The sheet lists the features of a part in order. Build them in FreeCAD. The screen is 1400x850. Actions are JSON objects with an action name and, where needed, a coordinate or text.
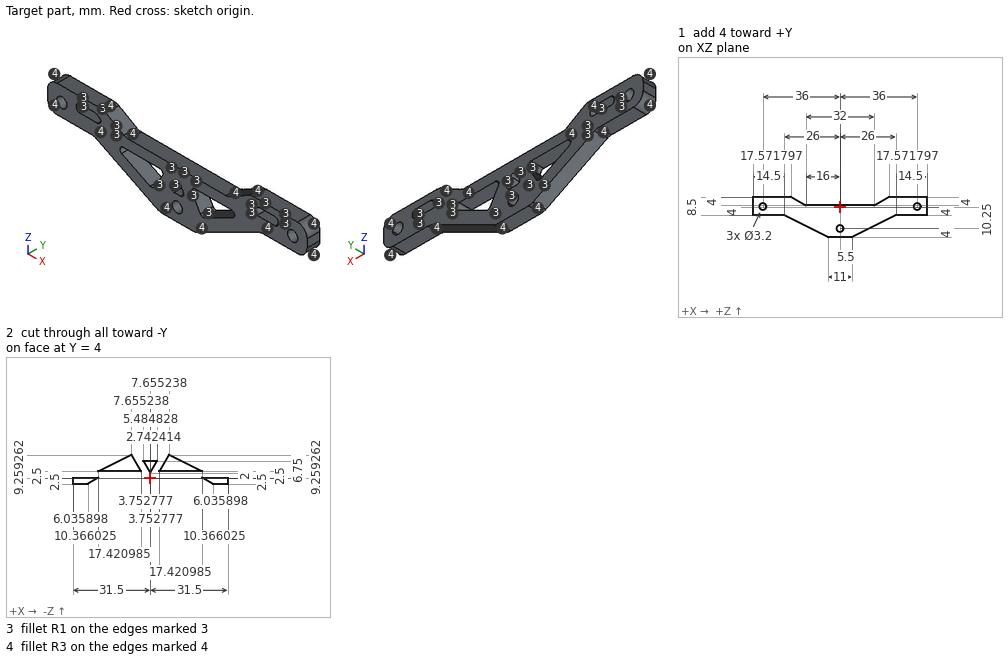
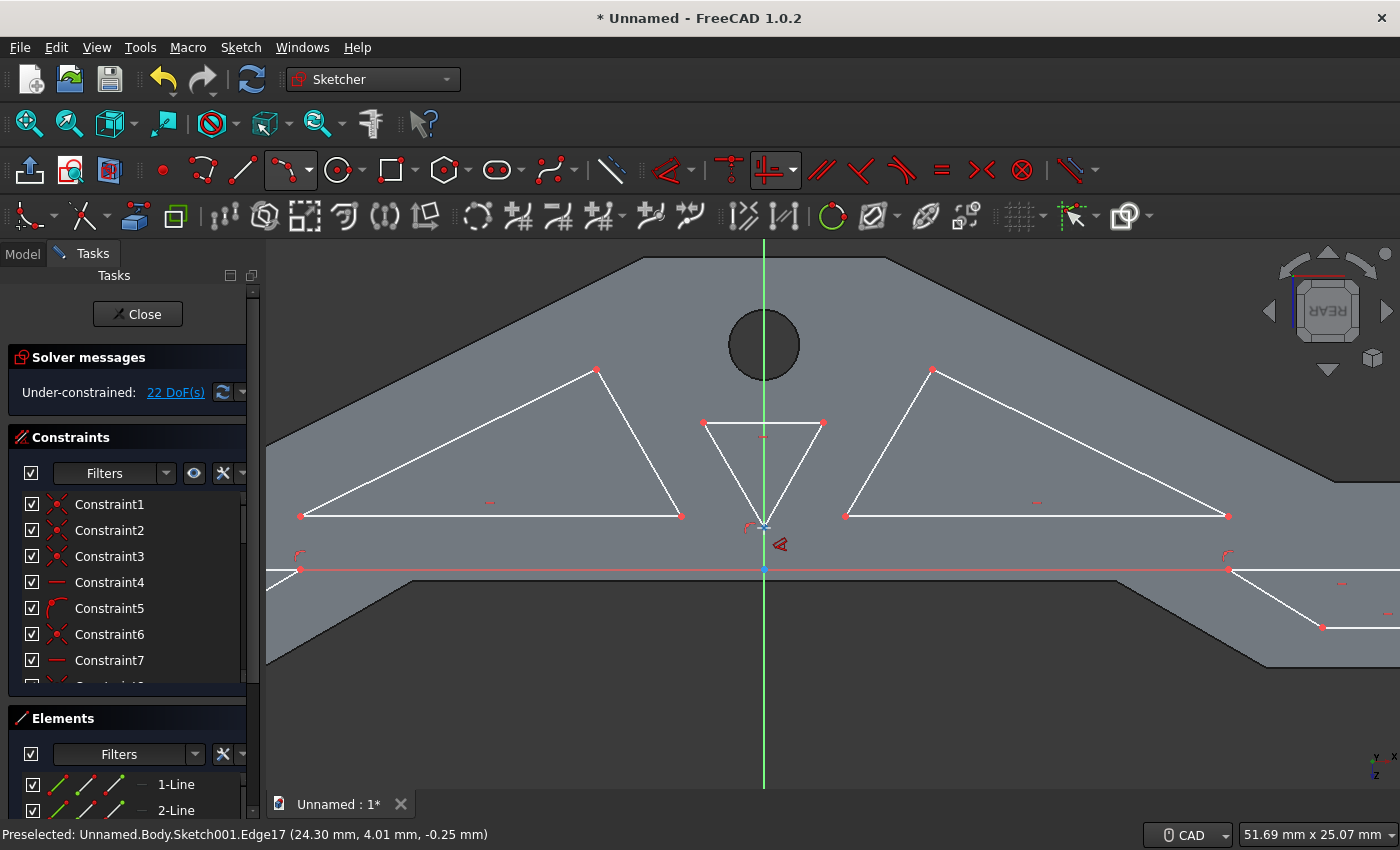
{"action": "left_click", "coordinate": [764, 527]}
{"action": "left_click", "coordinate": [798, 549]}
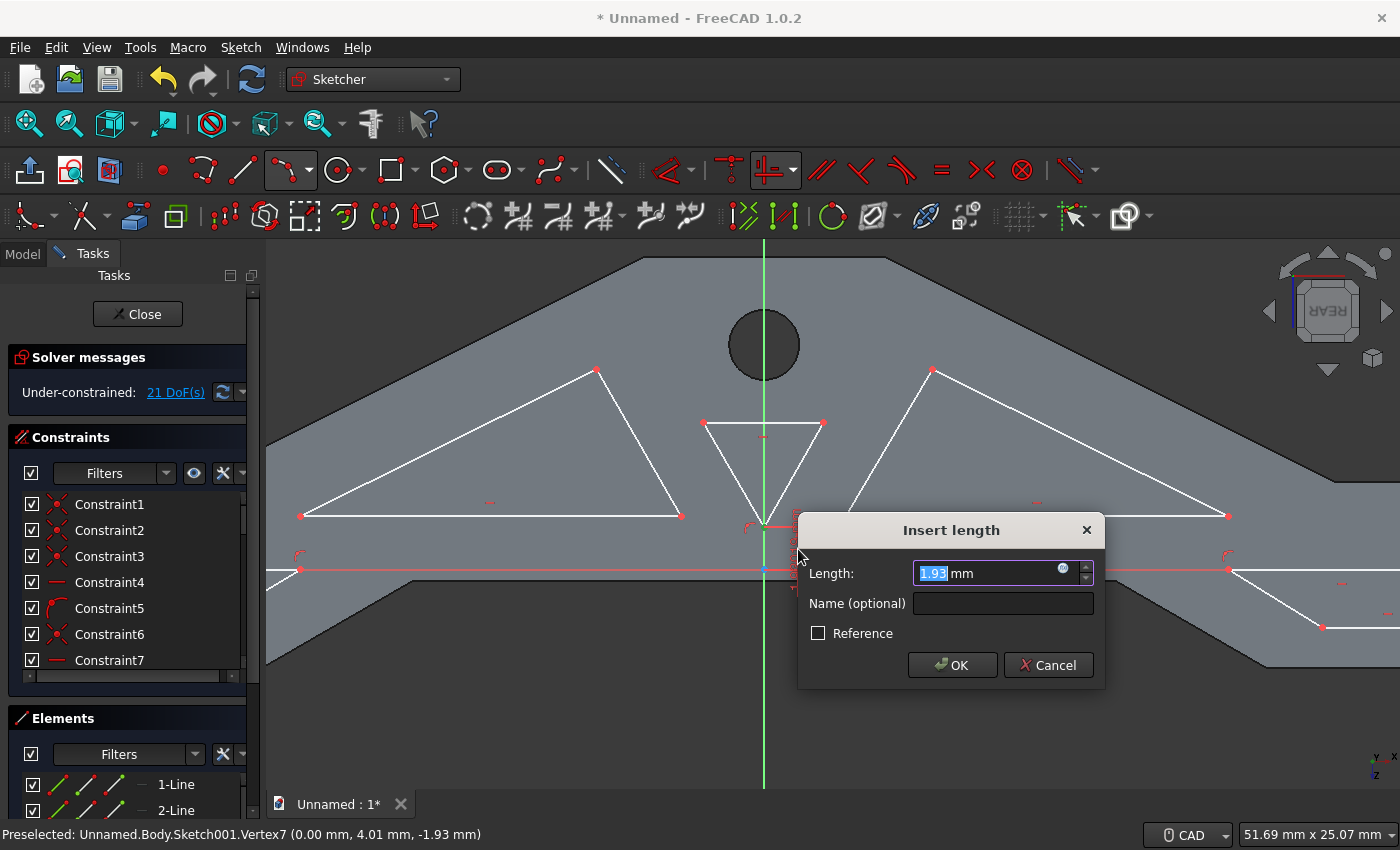
{"action": "type", "text": "2"}
{"action": "key", "text": "Return"}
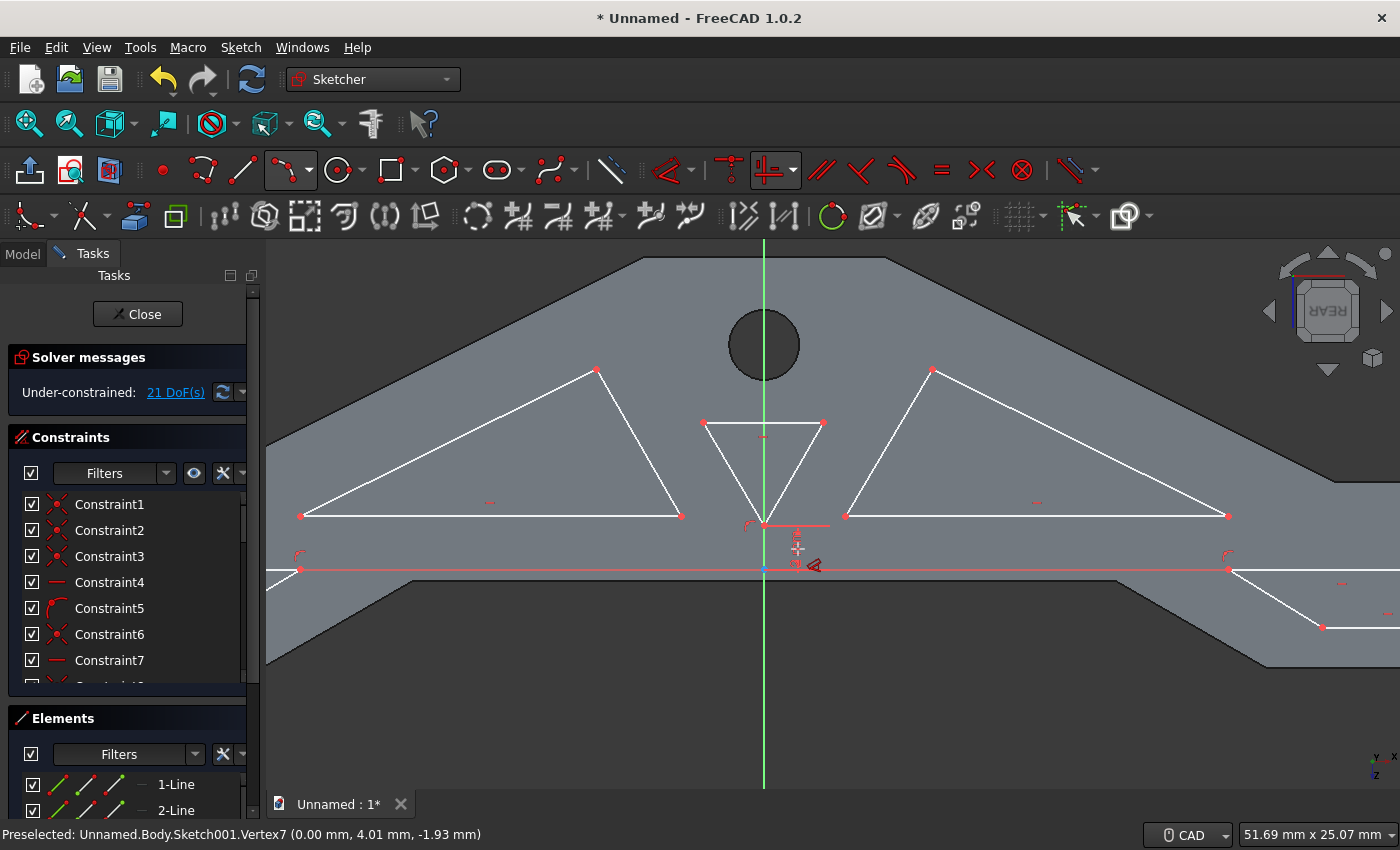
{"action": "scroll", "coordinate": [765, 529], "scroll_direction": "down", "scroll_amount": 4}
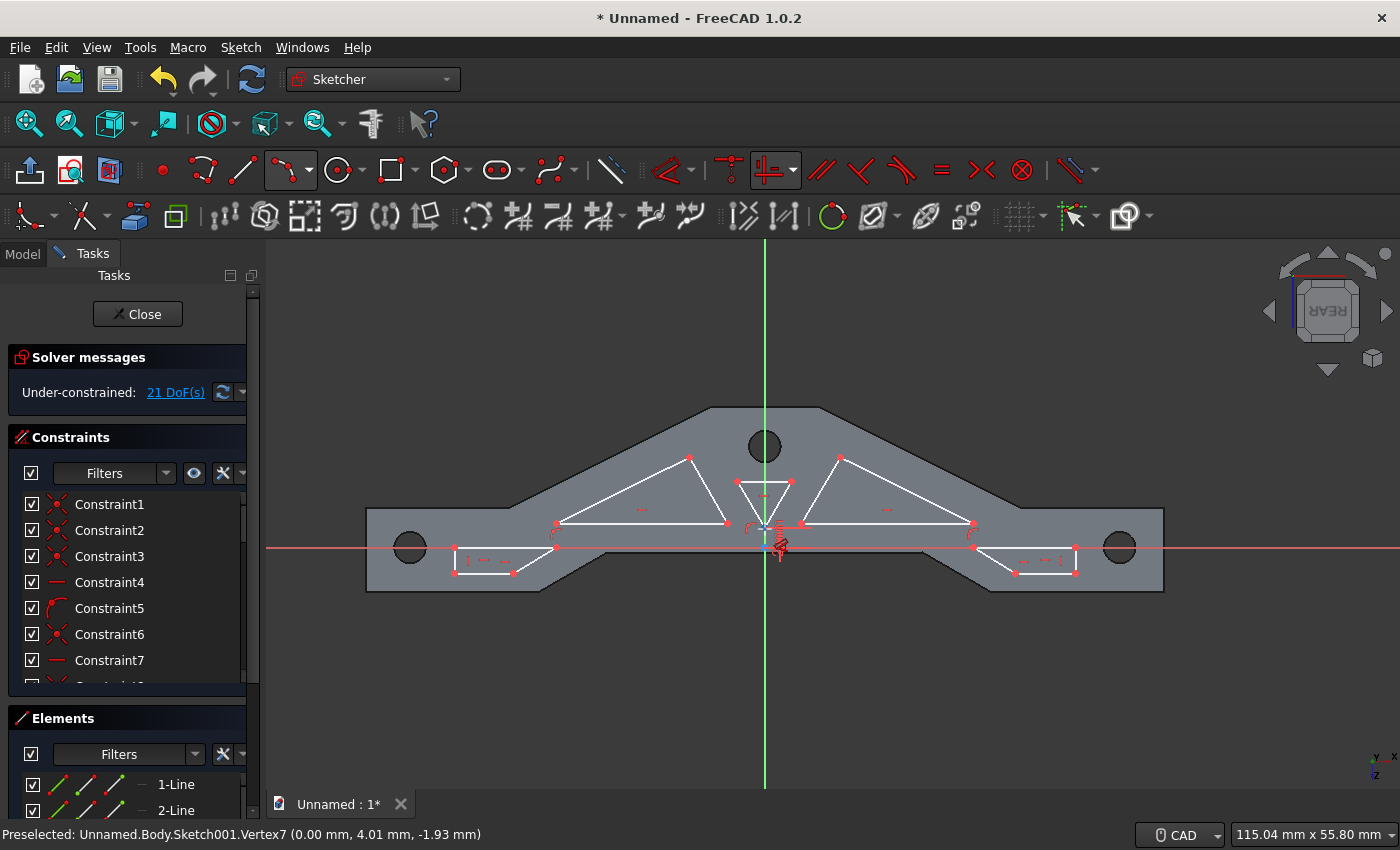
{"action": "scroll", "coordinate": [455, 555], "scroll_direction": "up", "scroll_amount": 3}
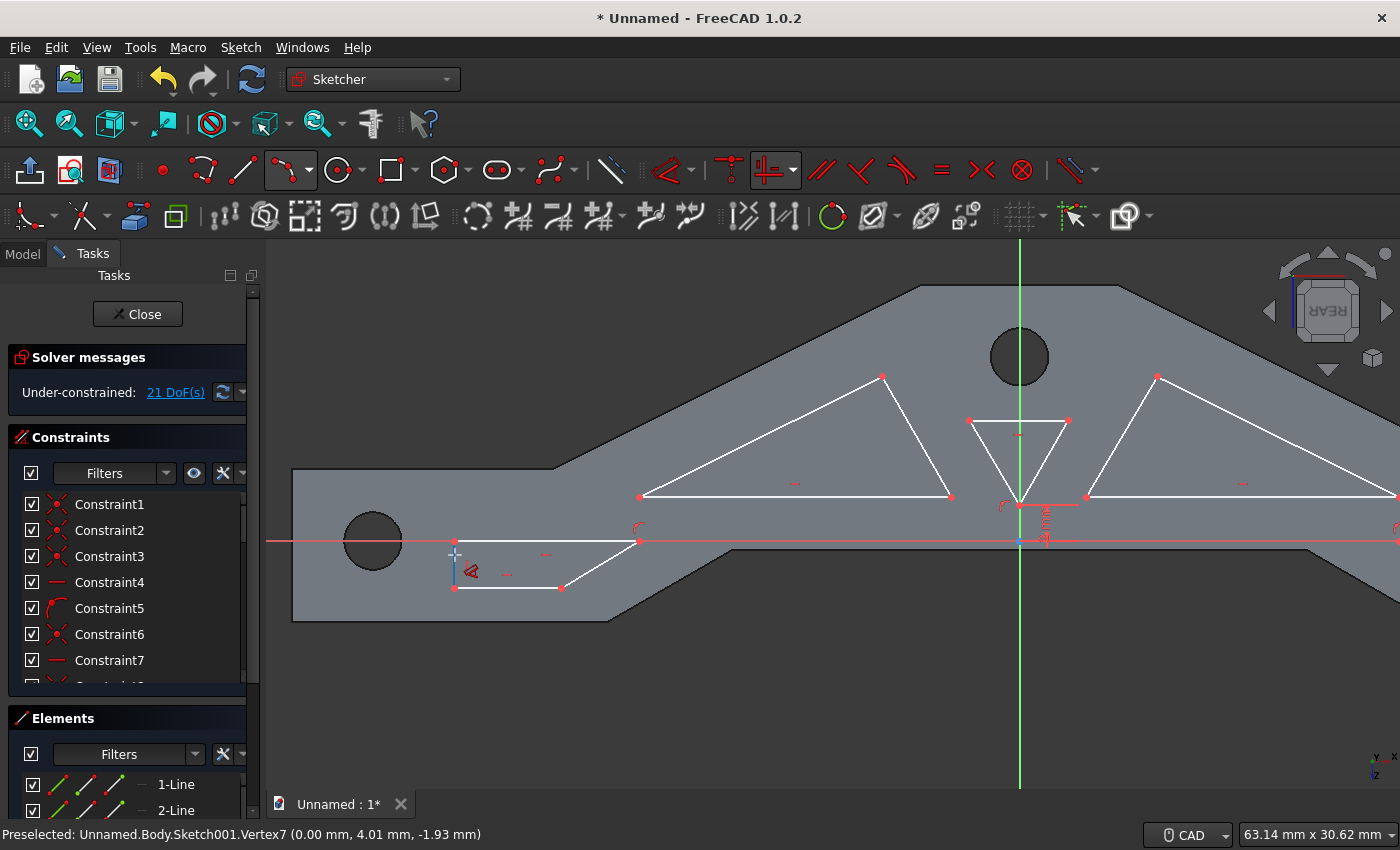
{"action": "left_click", "coordinate": [454, 555]}
{"action": "left_click", "coordinate": [420, 565]}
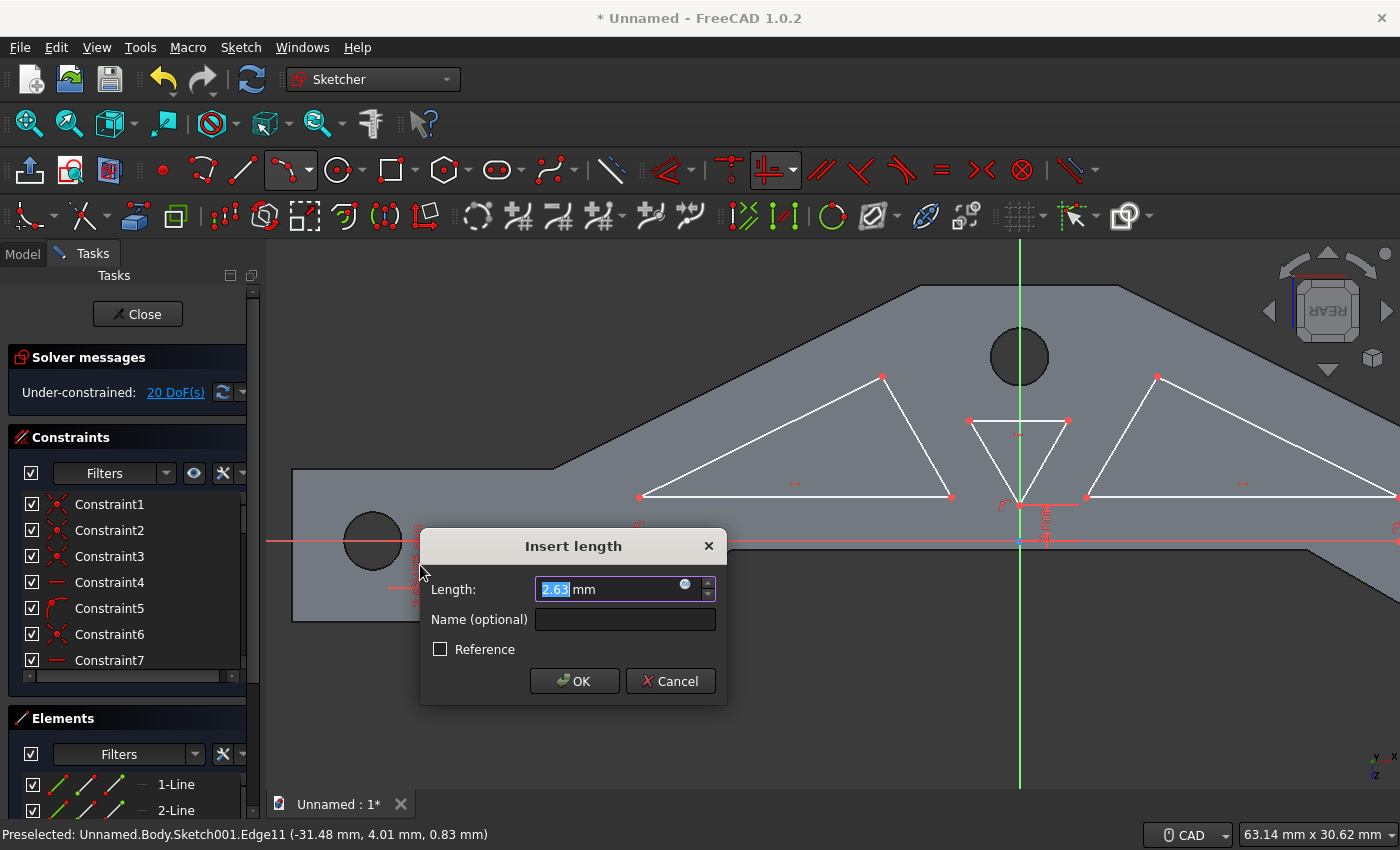
{"action": "type", "text": "2.5"}
{"action": "key", "text": "Return"}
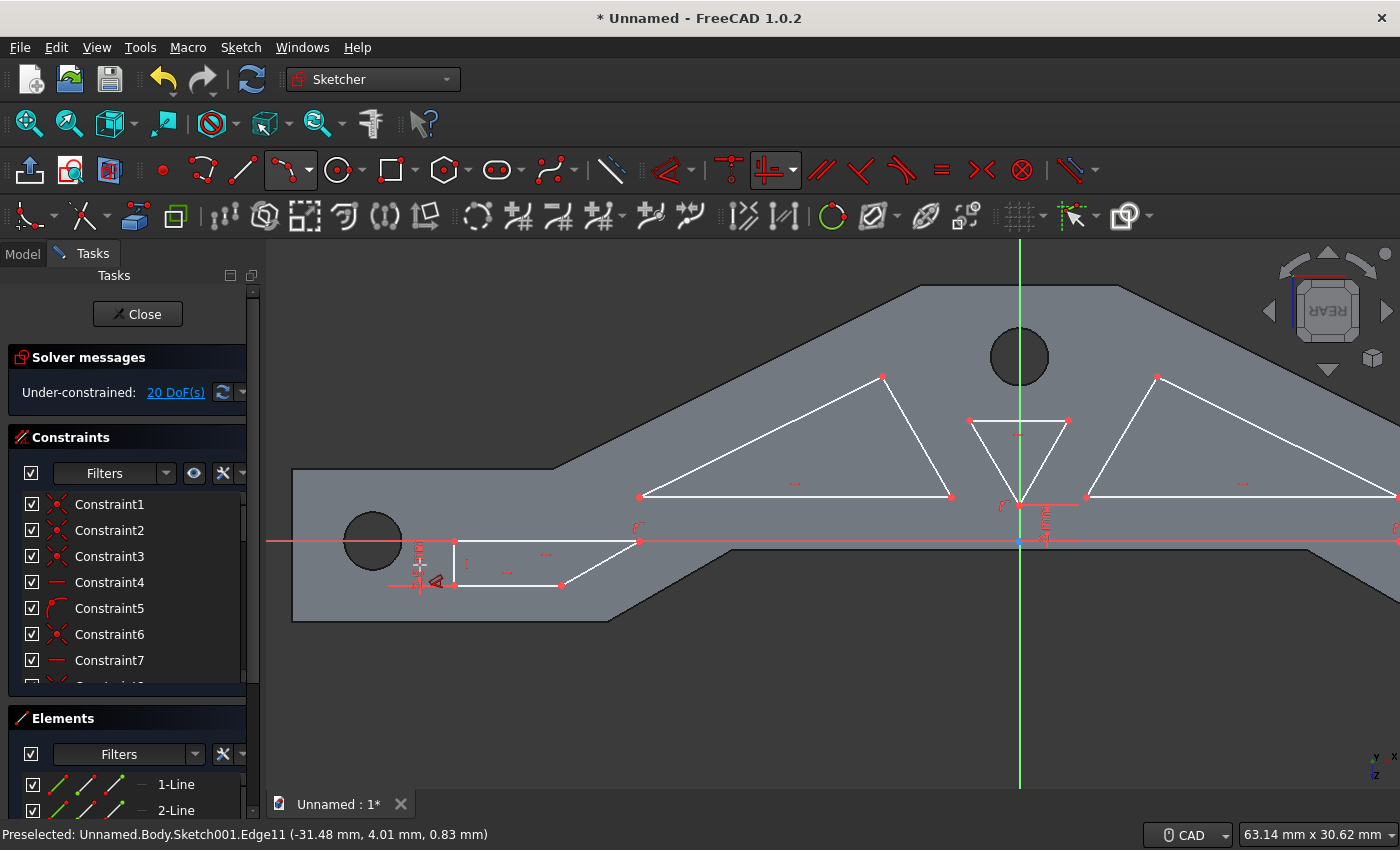
{"action": "scroll", "coordinate": [454, 555], "scroll_direction": "down", "scroll_amount": 3}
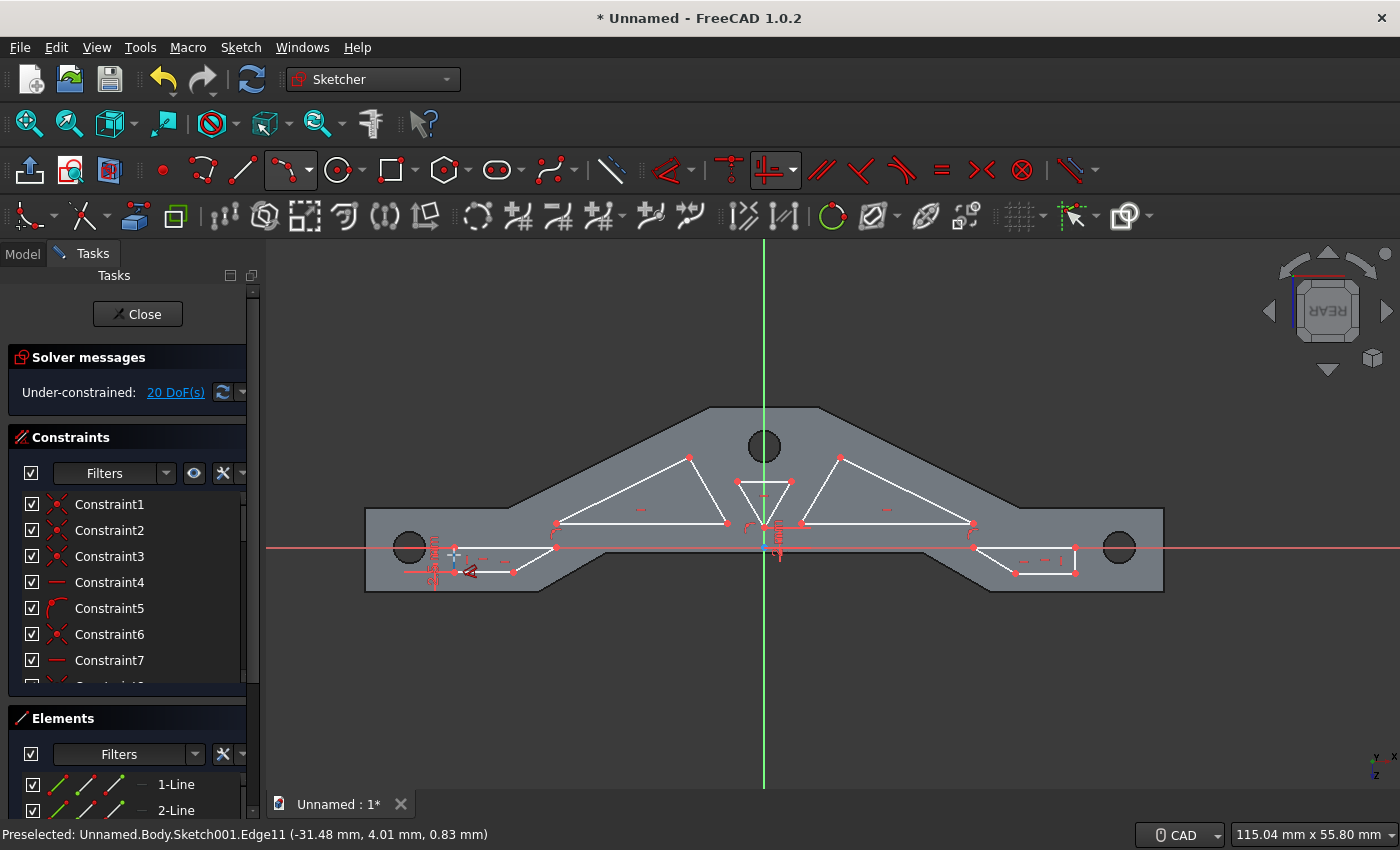
{"action": "scroll", "coordinate": [1075, 566], "scroll_direction": "up", "scroll_amount": 3}